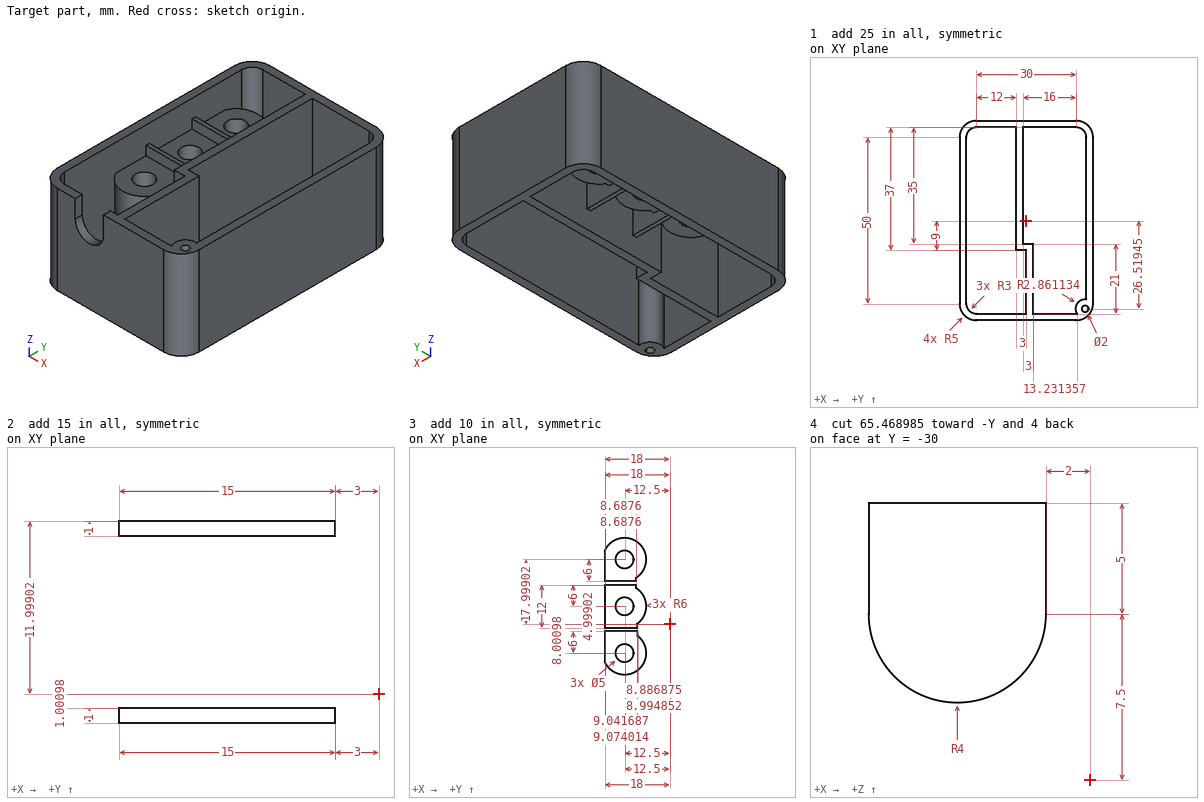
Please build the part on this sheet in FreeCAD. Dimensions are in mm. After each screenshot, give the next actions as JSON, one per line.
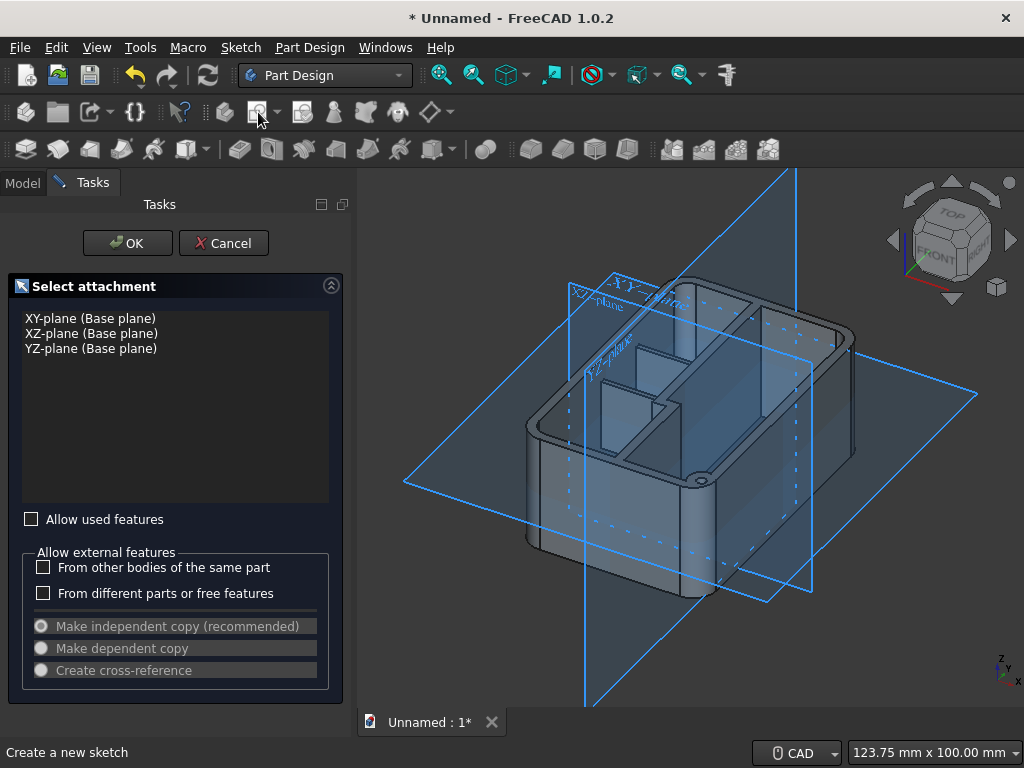
{"action": "left_click", "coordinate": [82, 318]}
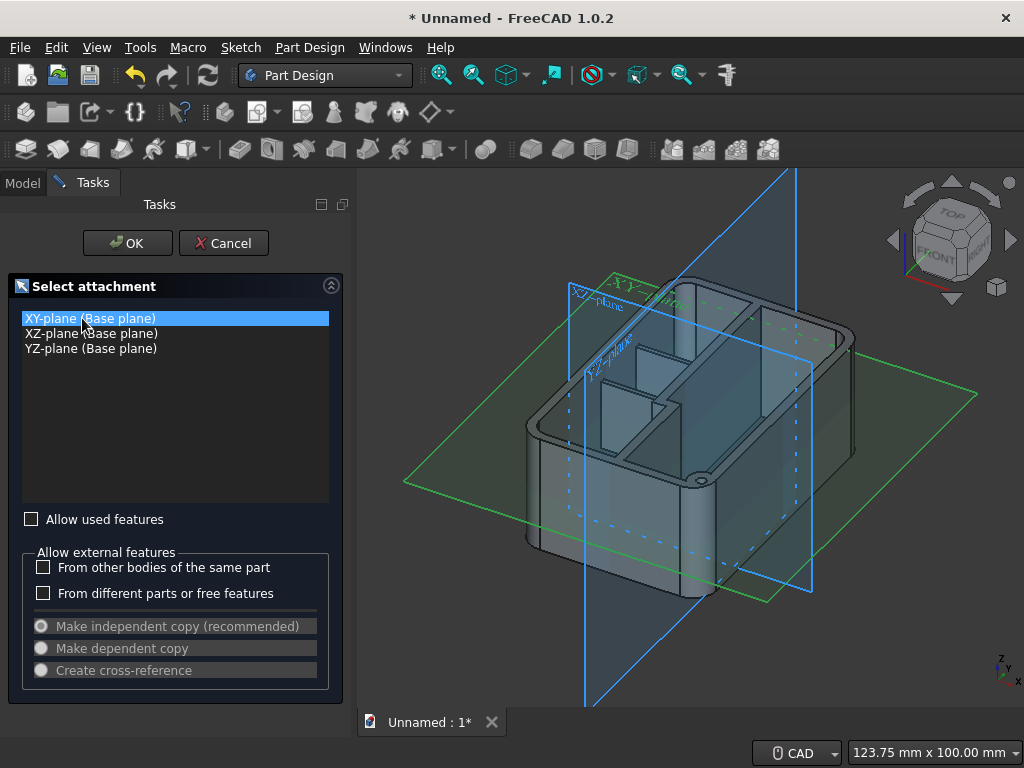
{"action": "left_click", "coordinate": [128, 243]}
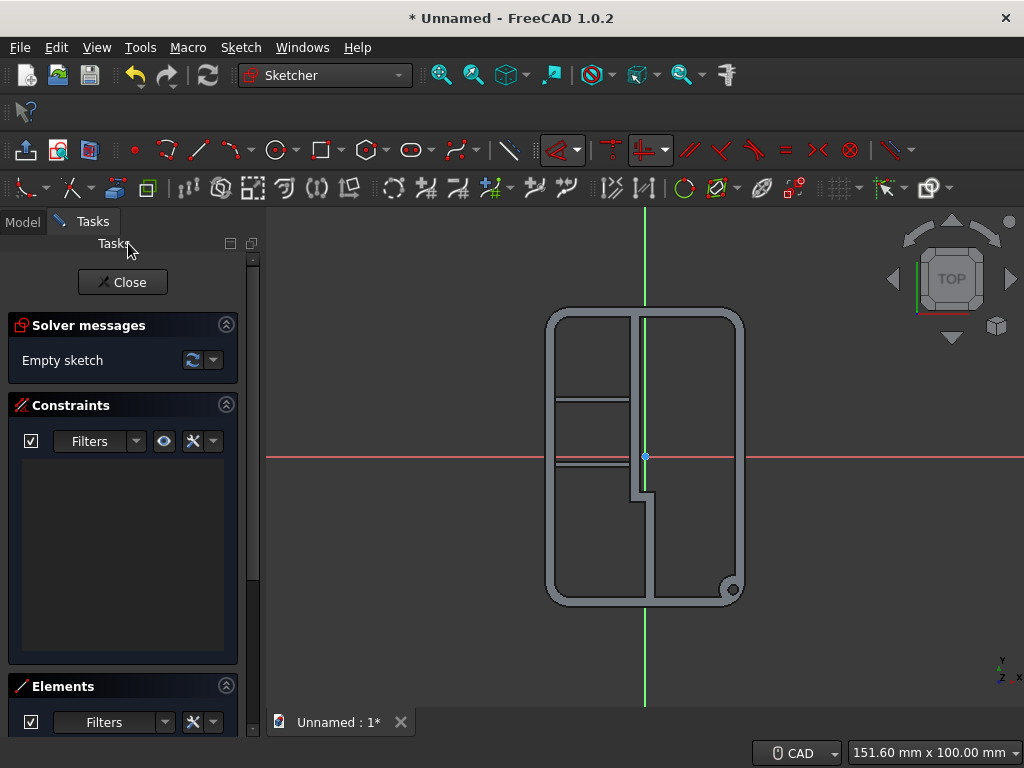
{"action": "left_click", "coordinate": [90, 150]}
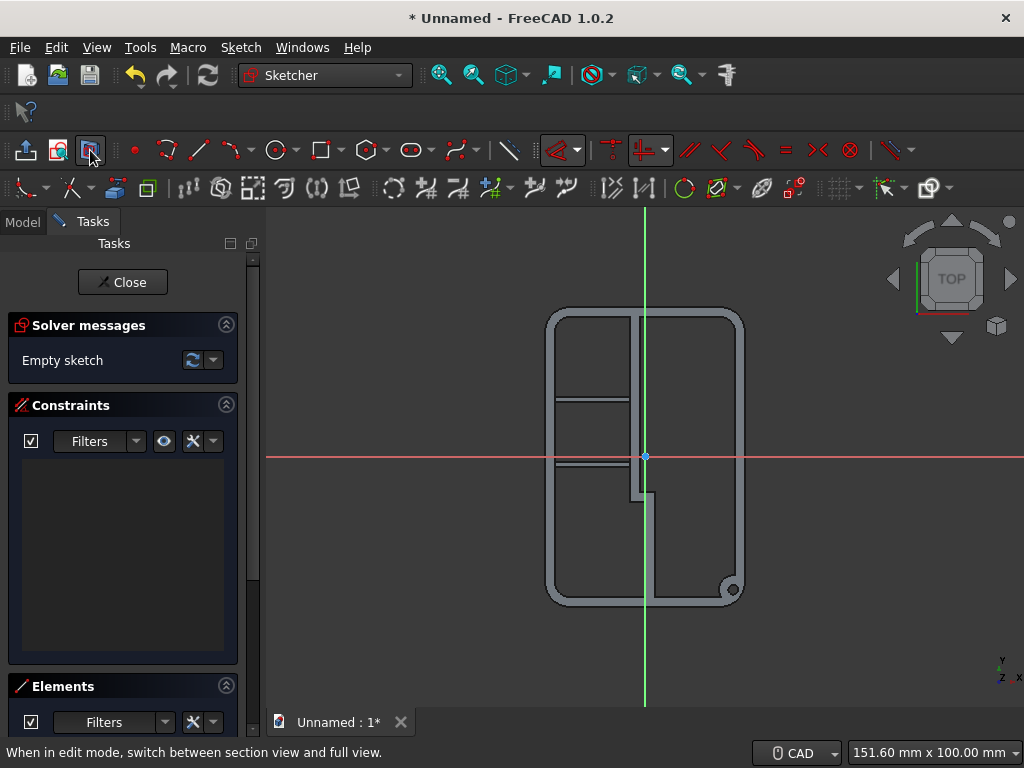
{"action": "scroll", "coordinate": [629, 403], "scroll_direction": "up", "scroll_amount": 3}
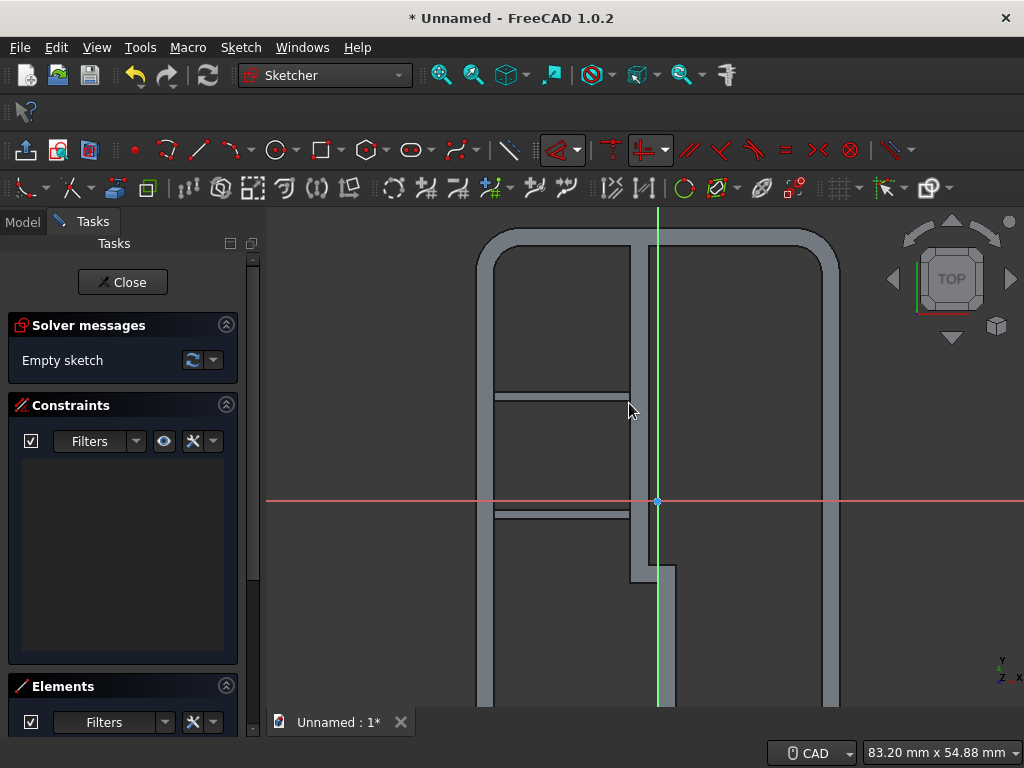
{"action": "left_click", "coordinate": [168, 150]}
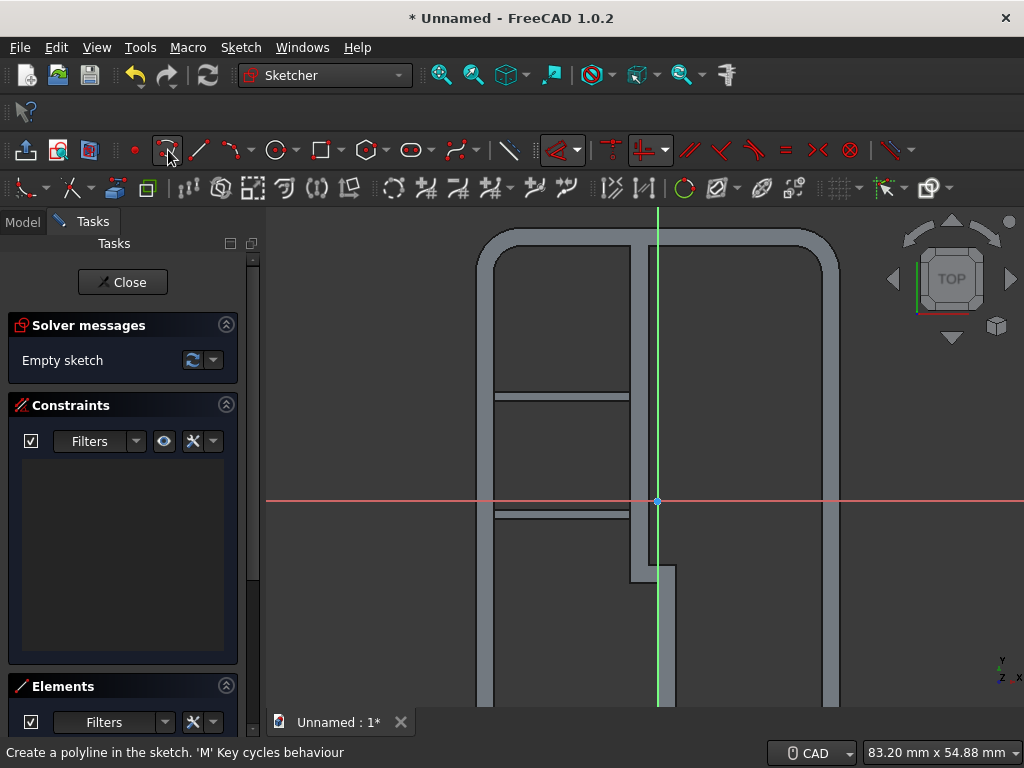
{"action": "left_click", "coordinate": [494, 315]}
{"action": "left_click", "coordinate": [494, 392]}
{"action": "left_click", "coordinate": [573, 392]}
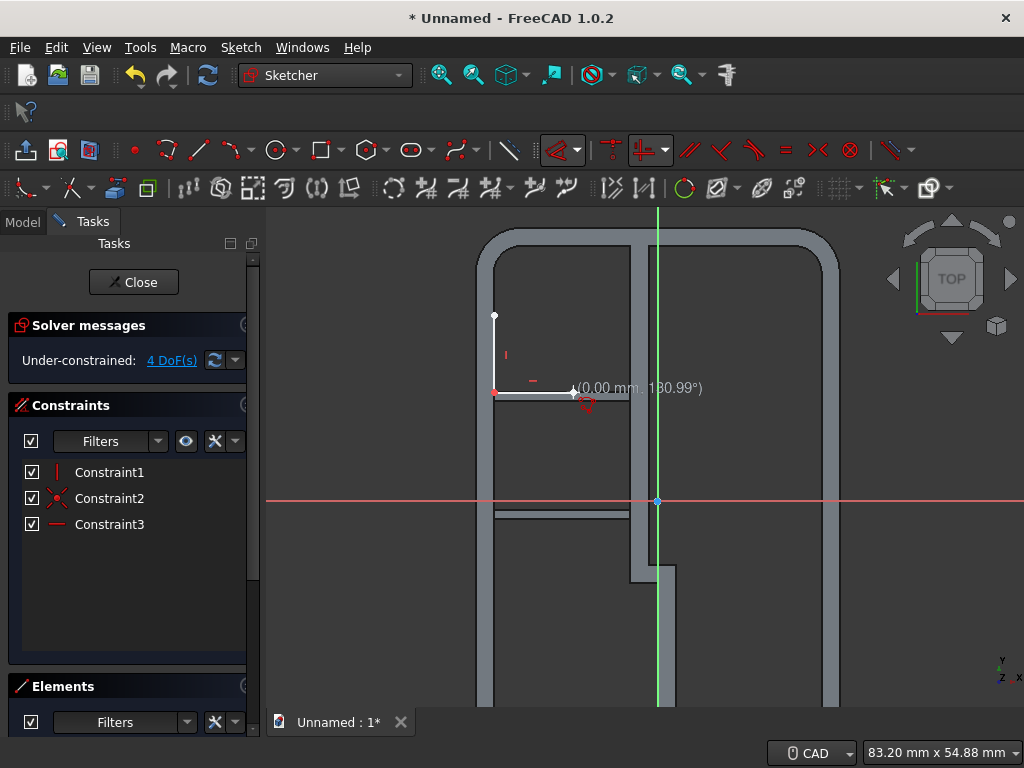
{"action": "scroll", "coordinate": [573, 383], "scroll_direction": "up", "scroll_amount": 4}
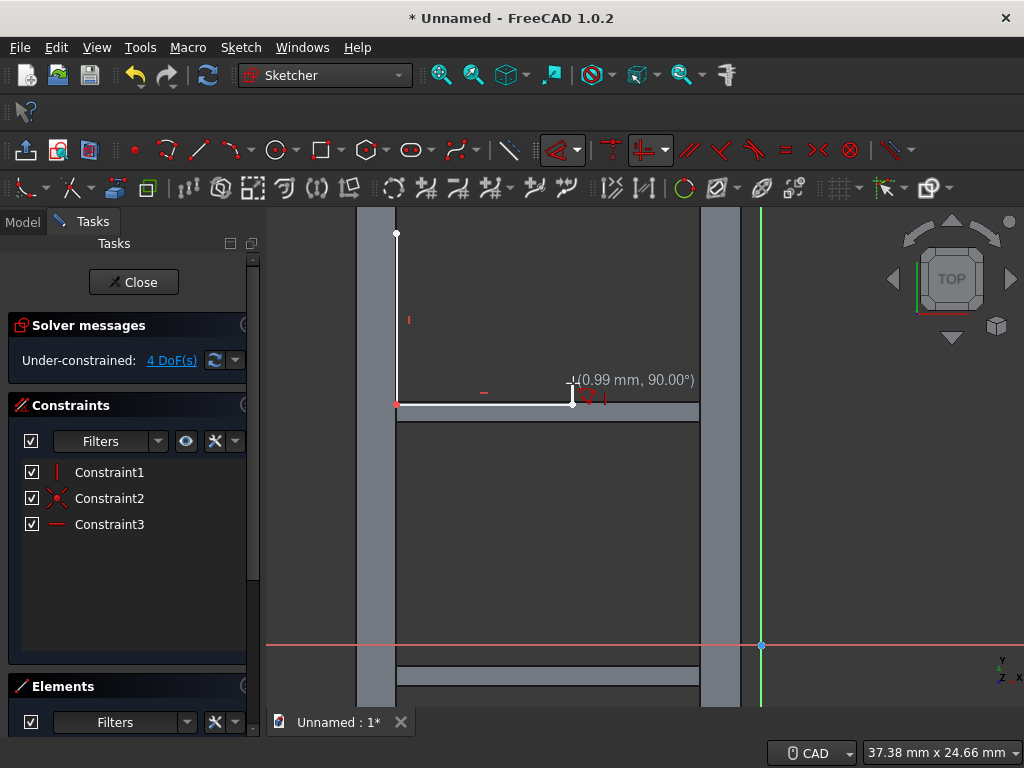
{"action": "left_click", "coordinate": [573, 383]}
{"action": "right_click", "coordinate": [573, 383]}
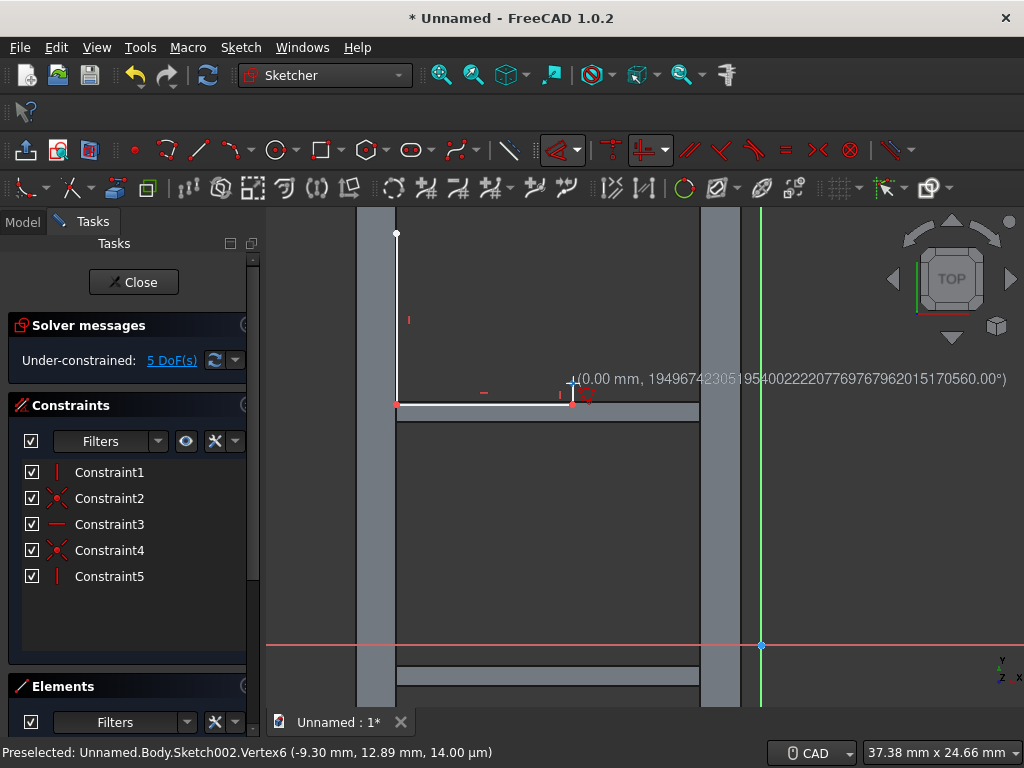
{"action": "left_click", "coordinate": [232, 150]}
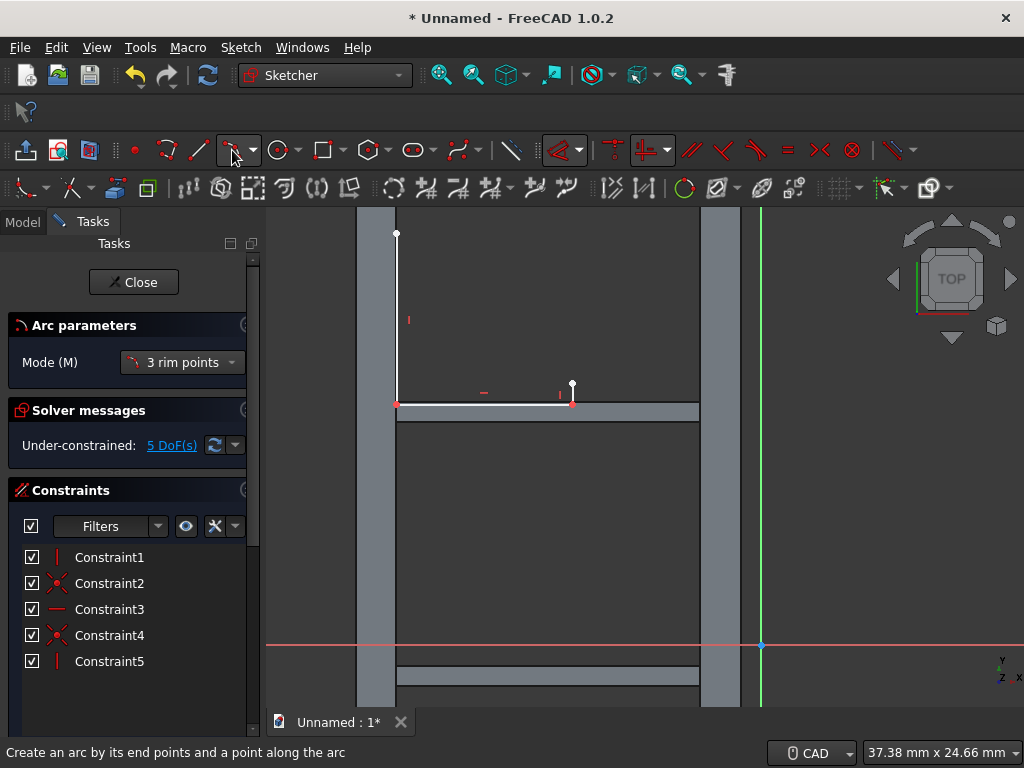
{"action": "scroll", "coordinate": [572, 383], "scroll_direction": "up", "scroll_amount": 3}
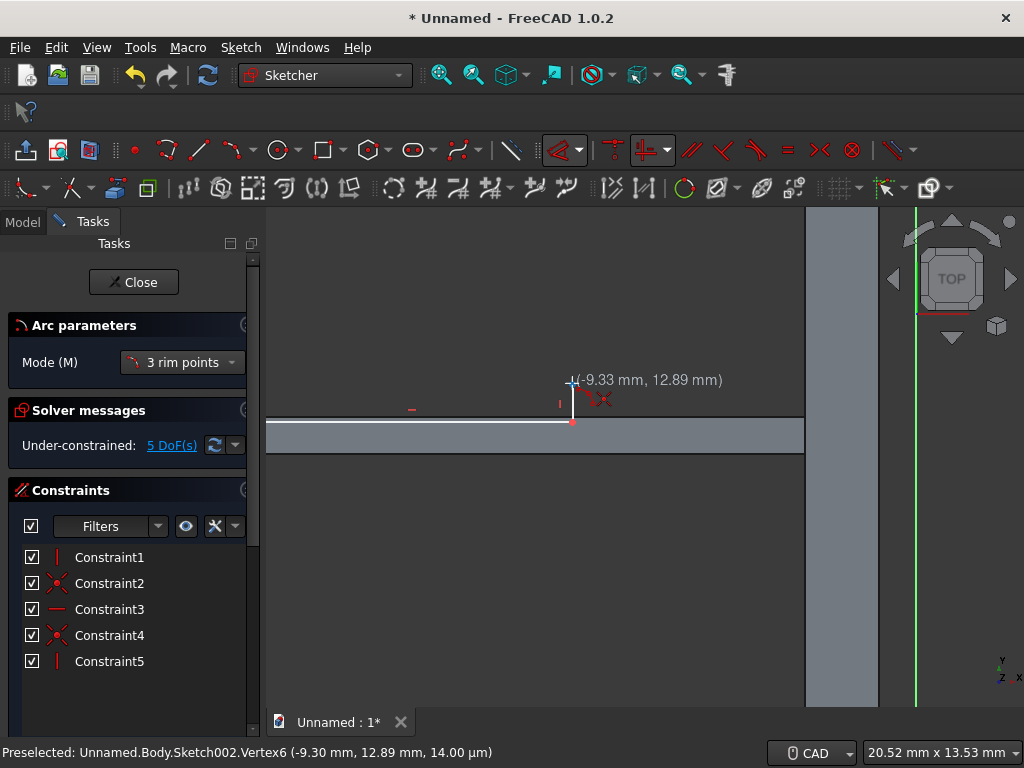
{"action": "left_click", "coordinate": [573, 385]}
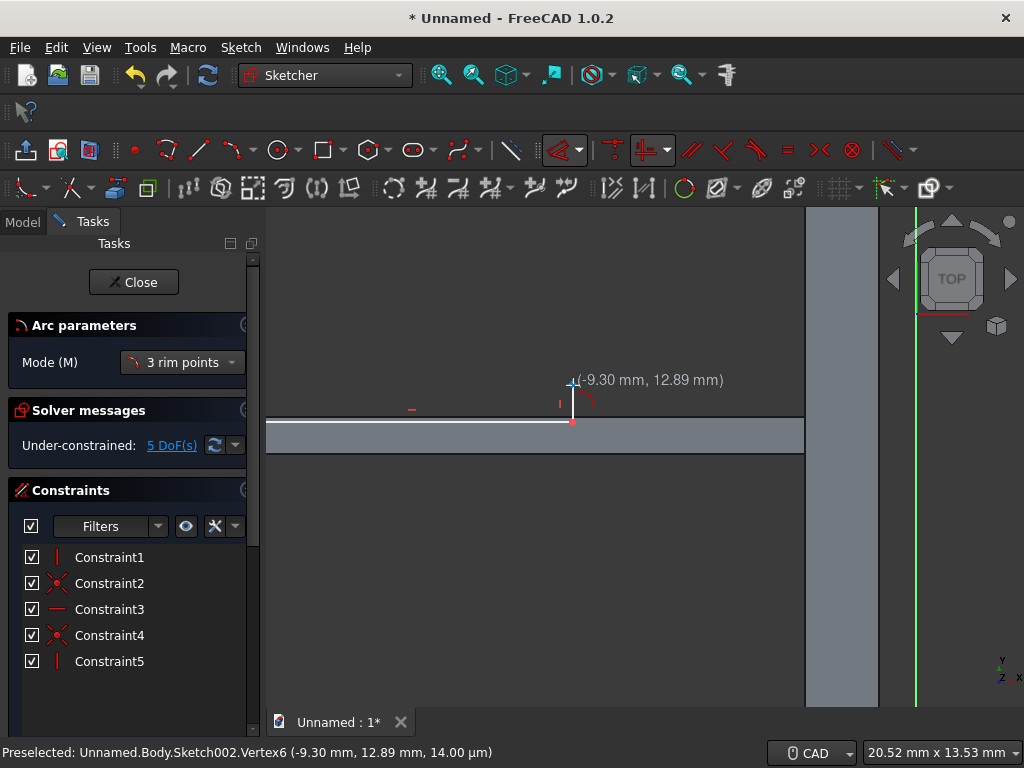
{"action": "scroll", "coordinate": [574, 384], "scroll_direction": "down", "scroll_amount": 7}